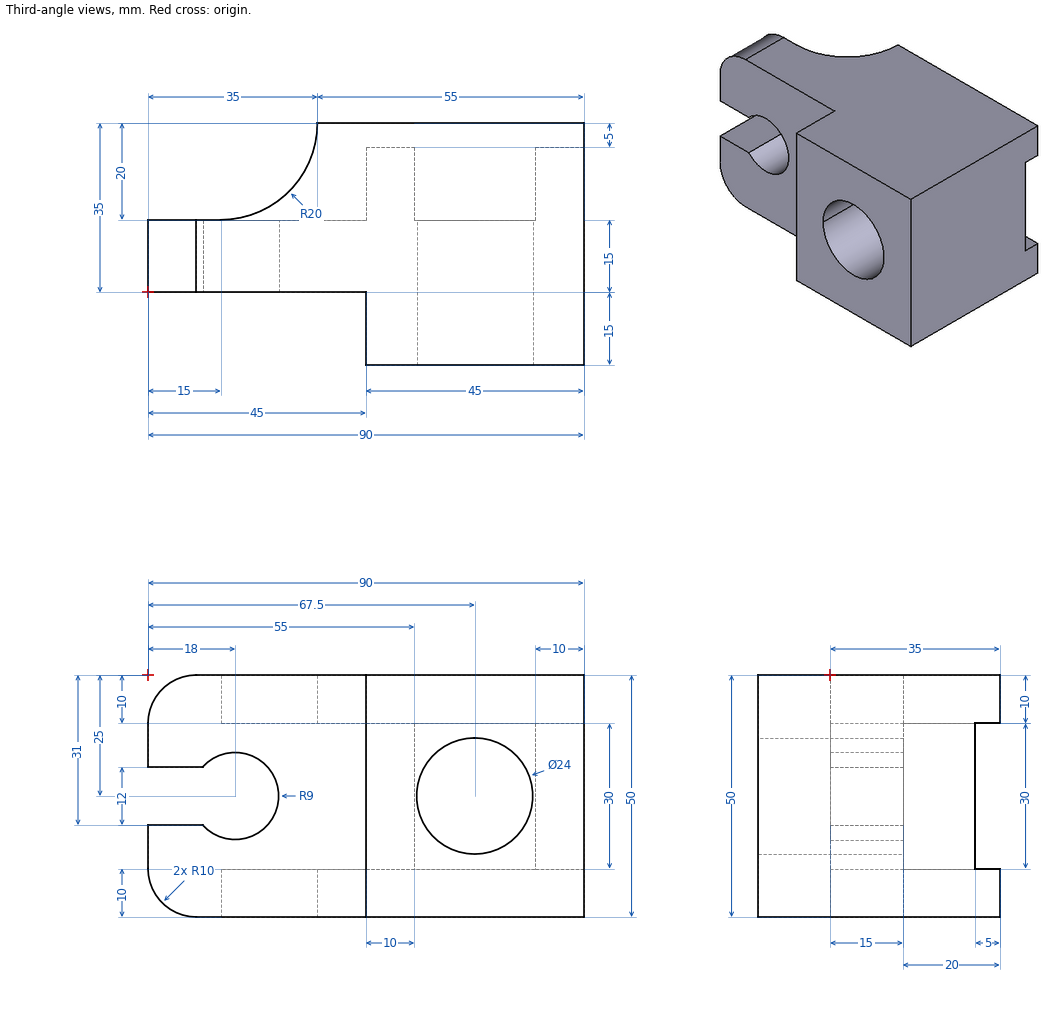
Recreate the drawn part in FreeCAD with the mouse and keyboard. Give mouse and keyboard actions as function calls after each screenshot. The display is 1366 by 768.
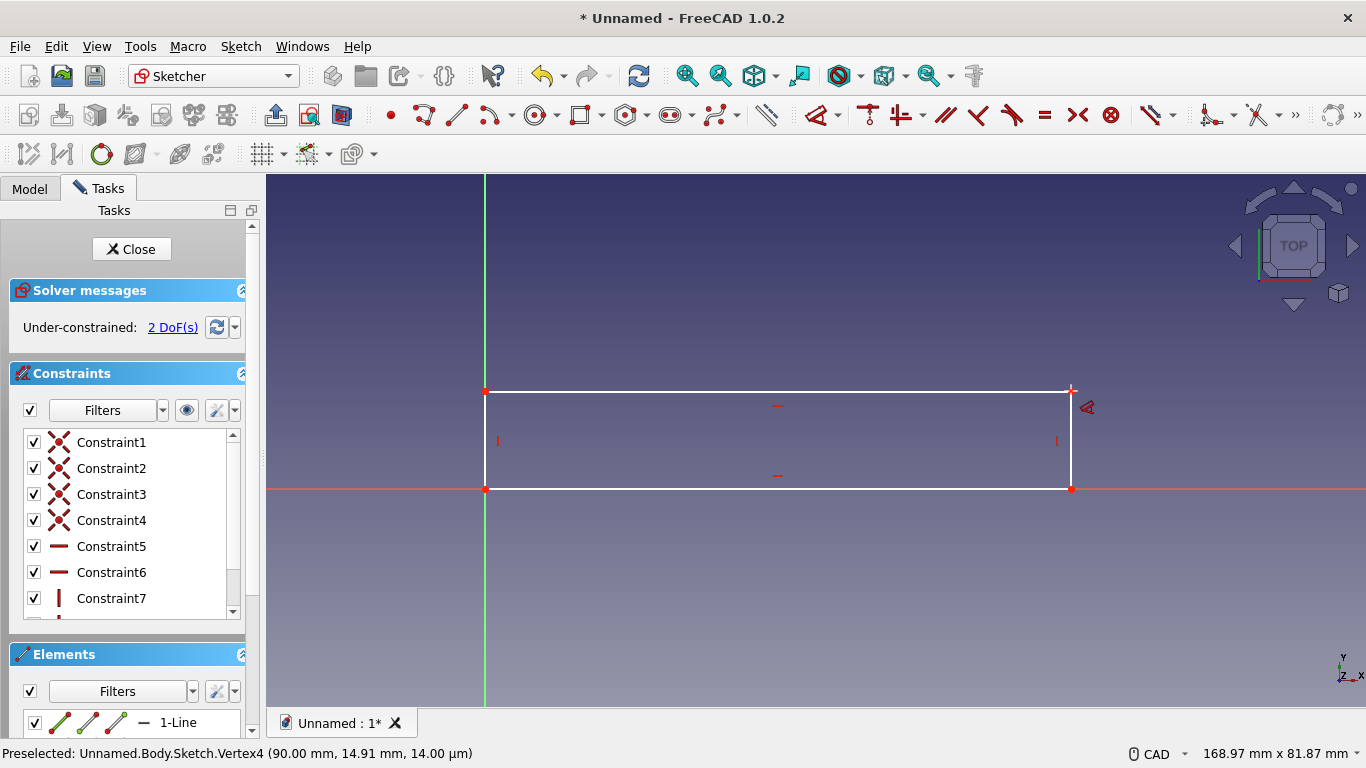
click(661, 489)
click(778, 523)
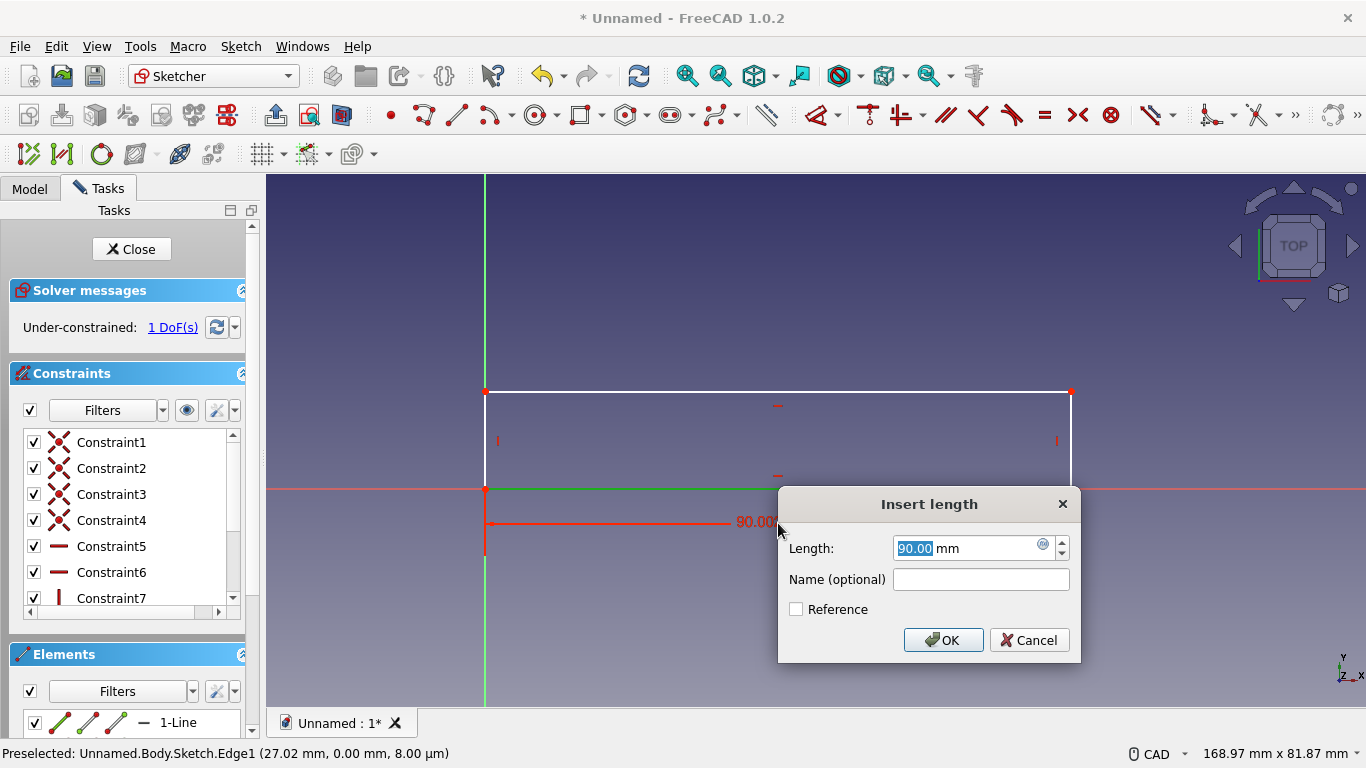
text(90)
key(Return)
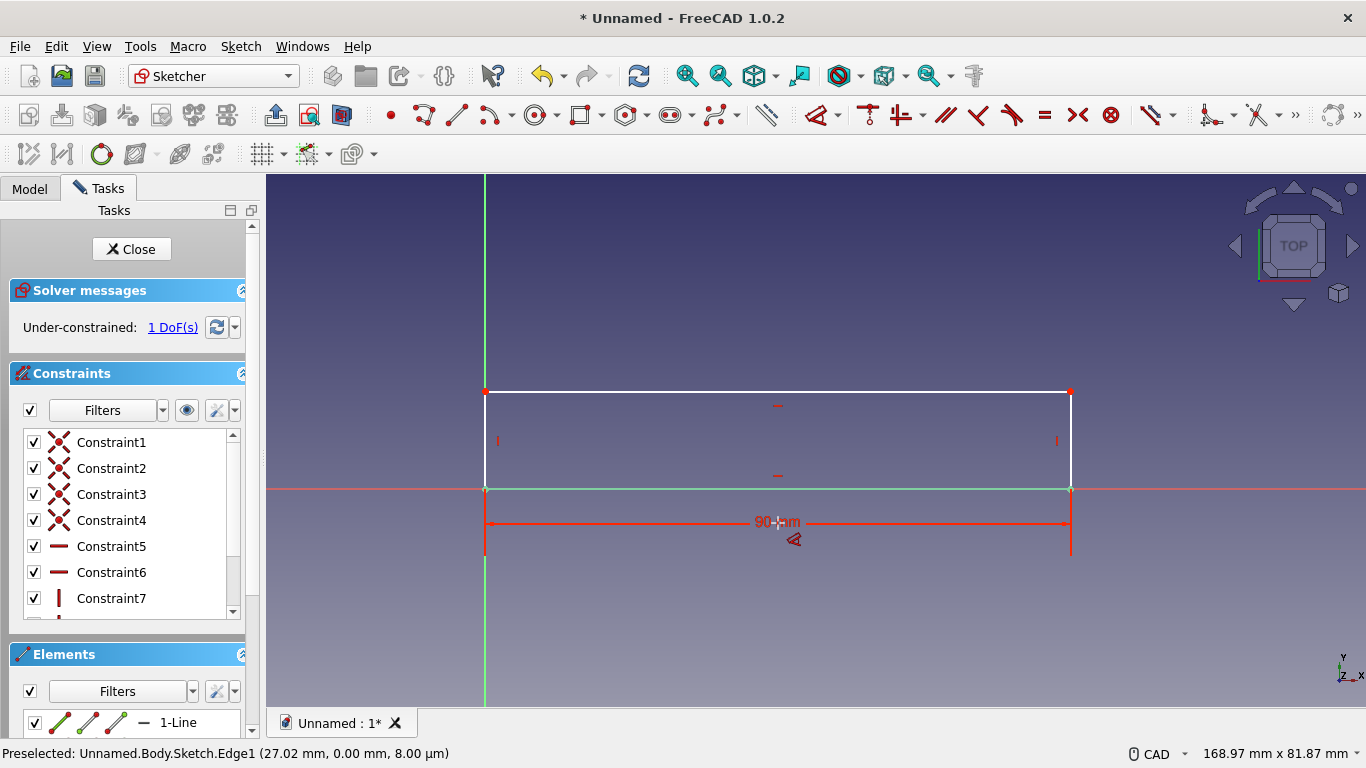
click(1071, 460)
click(1105, 441)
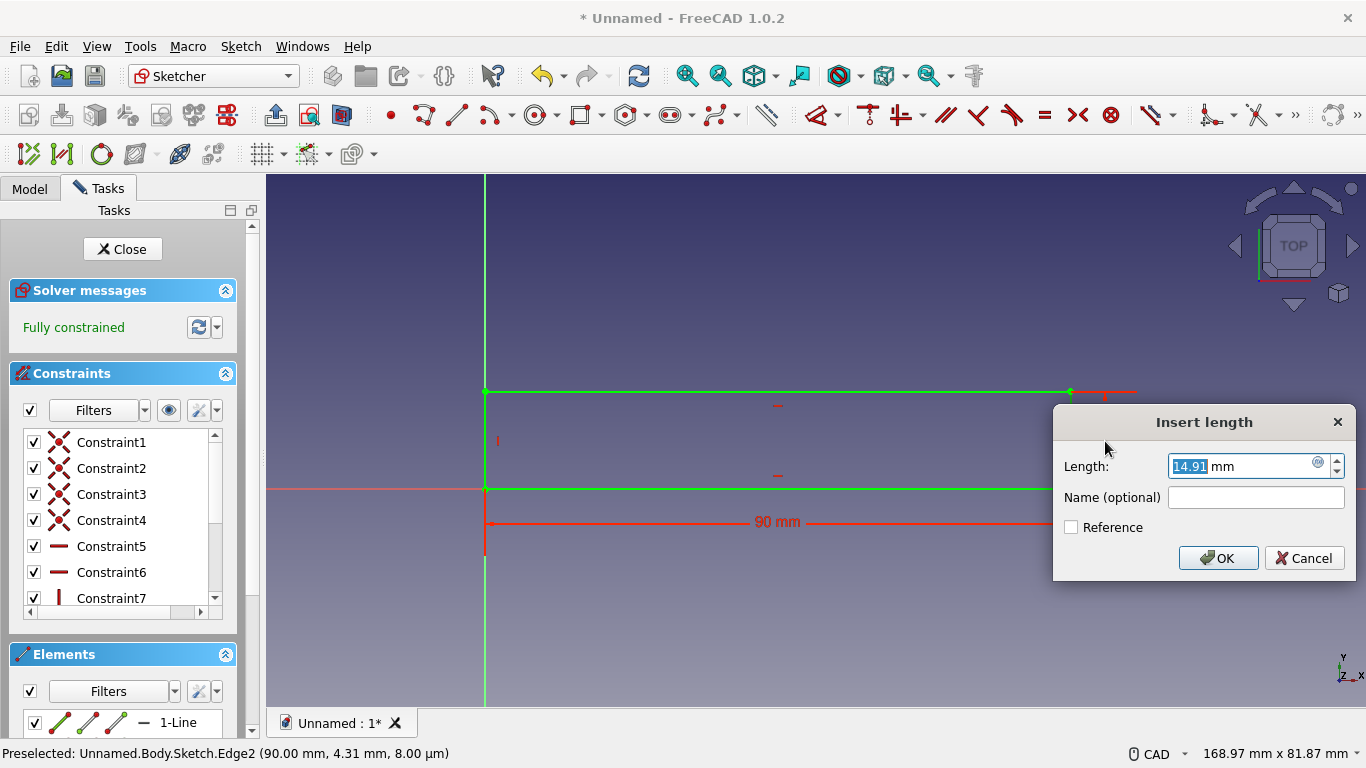
text(15)
key(Return)
key(Escape)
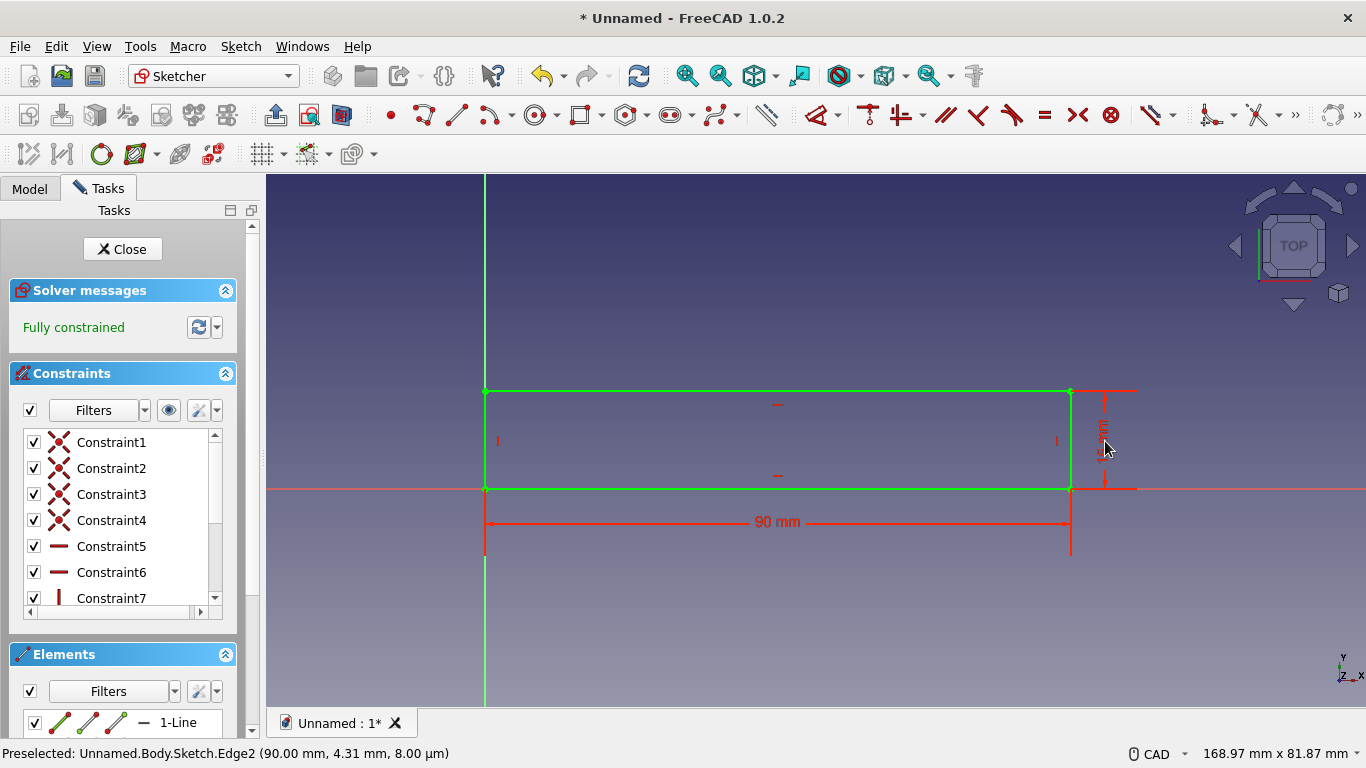
click(123, 249)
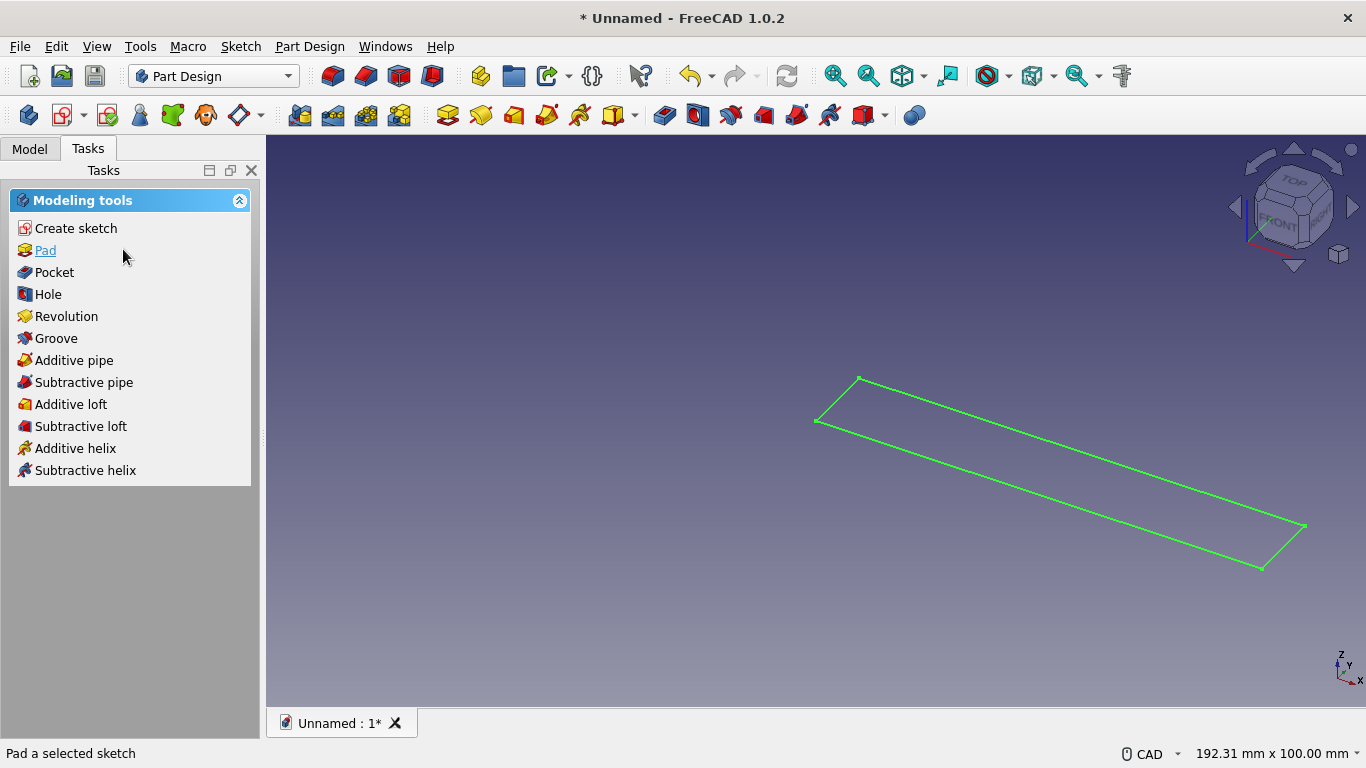
click(448, 116)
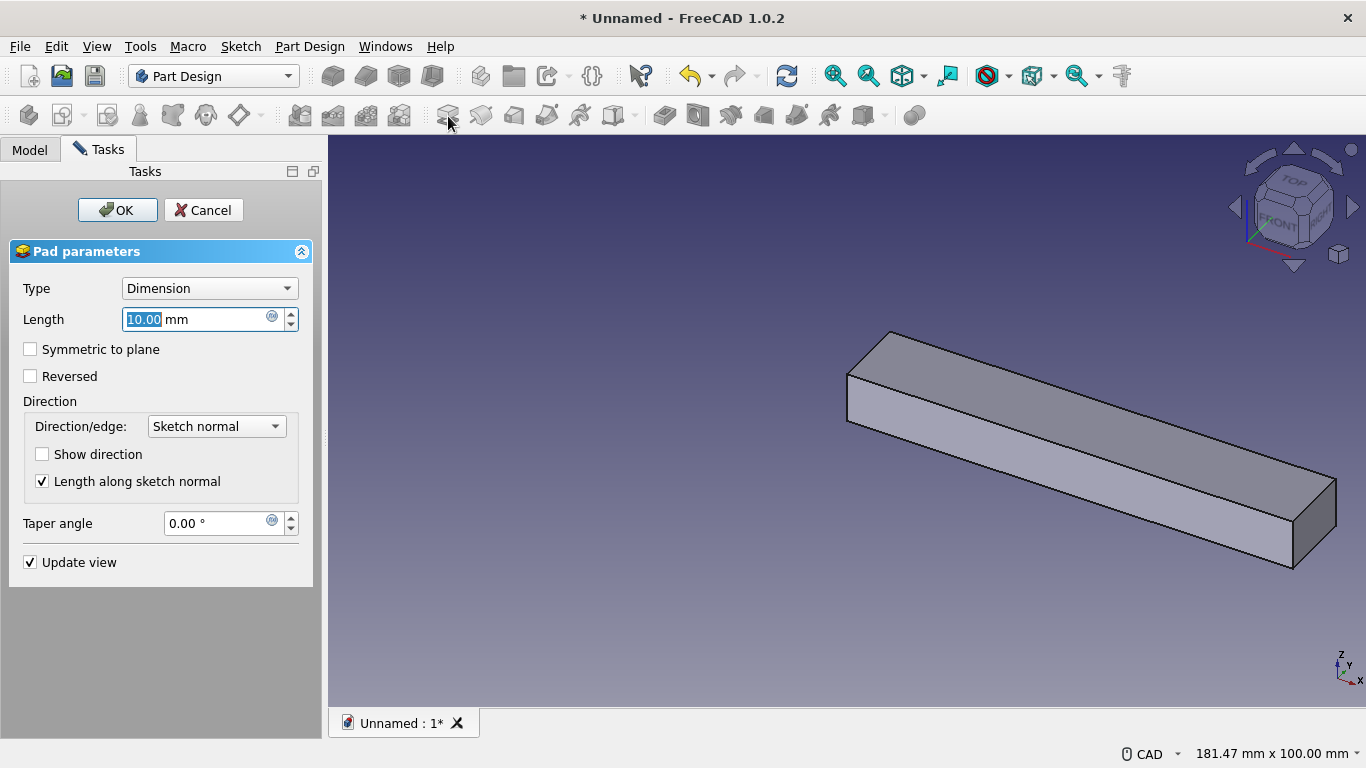
text(50)
key(Tab)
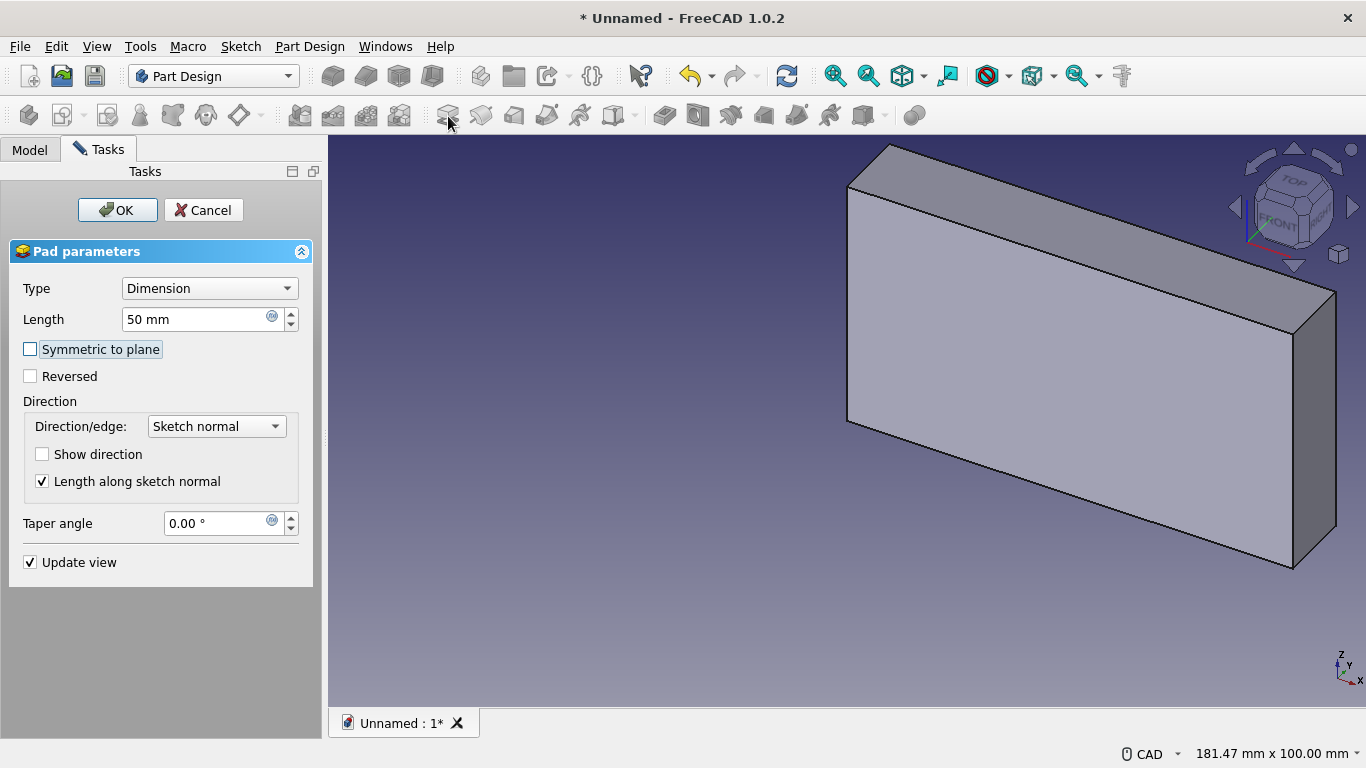
click(31, 376)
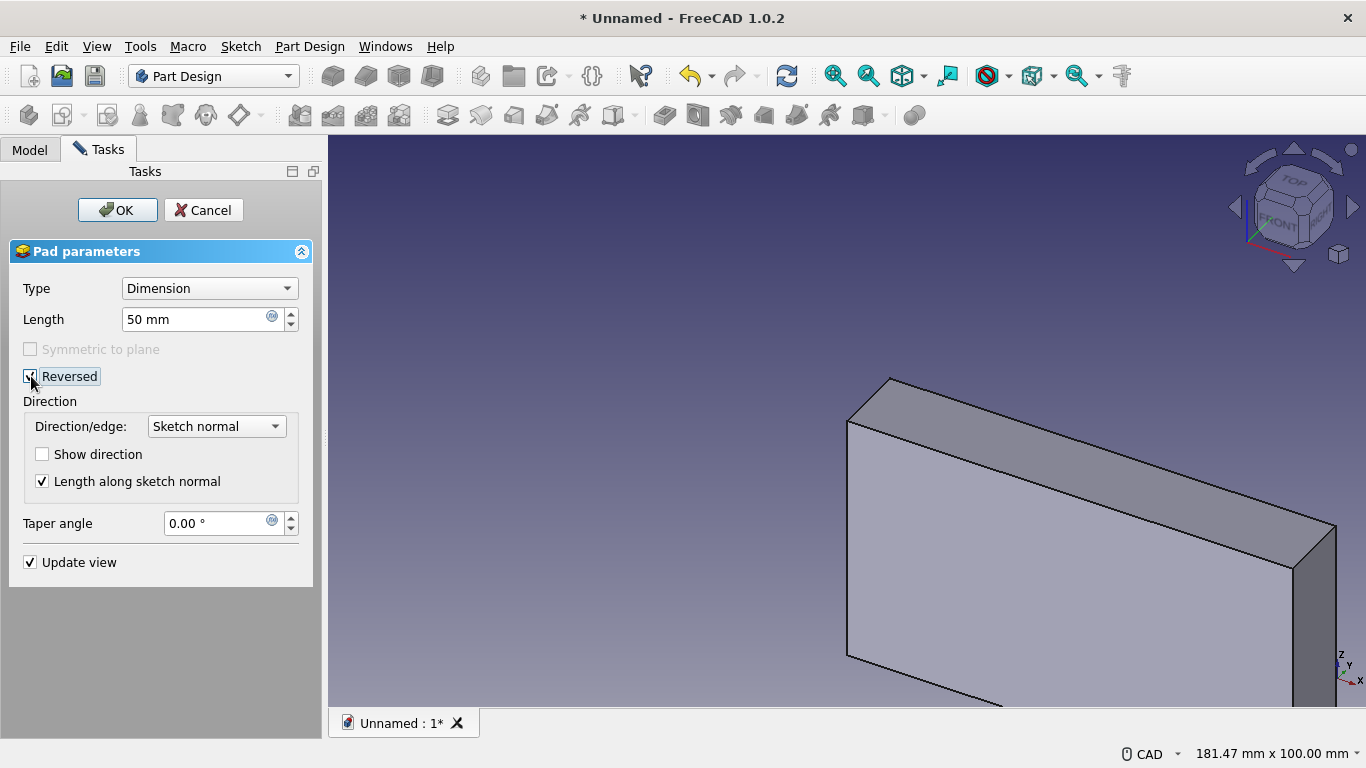
click(118, 210)